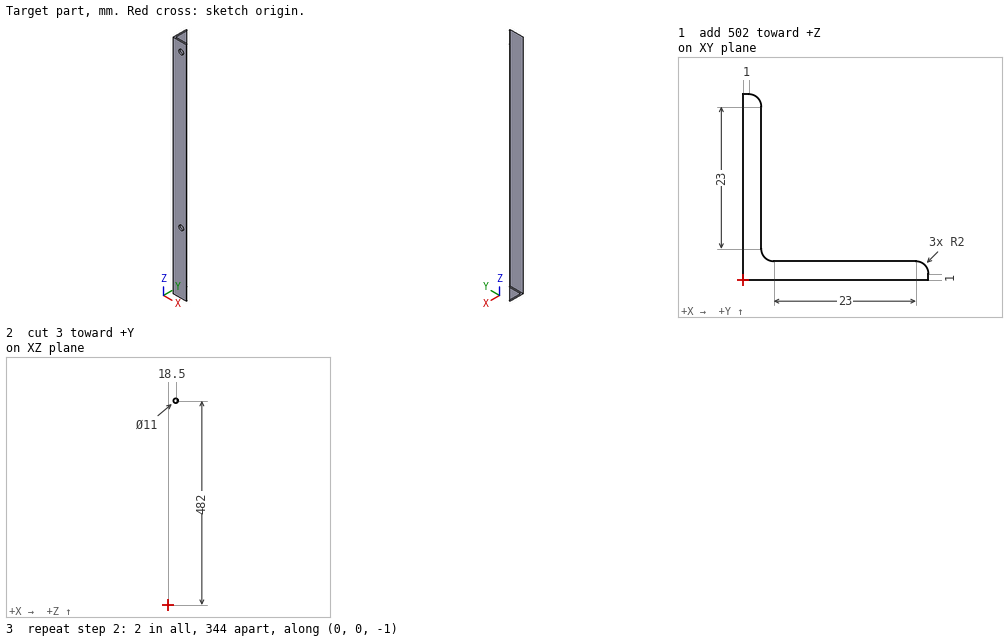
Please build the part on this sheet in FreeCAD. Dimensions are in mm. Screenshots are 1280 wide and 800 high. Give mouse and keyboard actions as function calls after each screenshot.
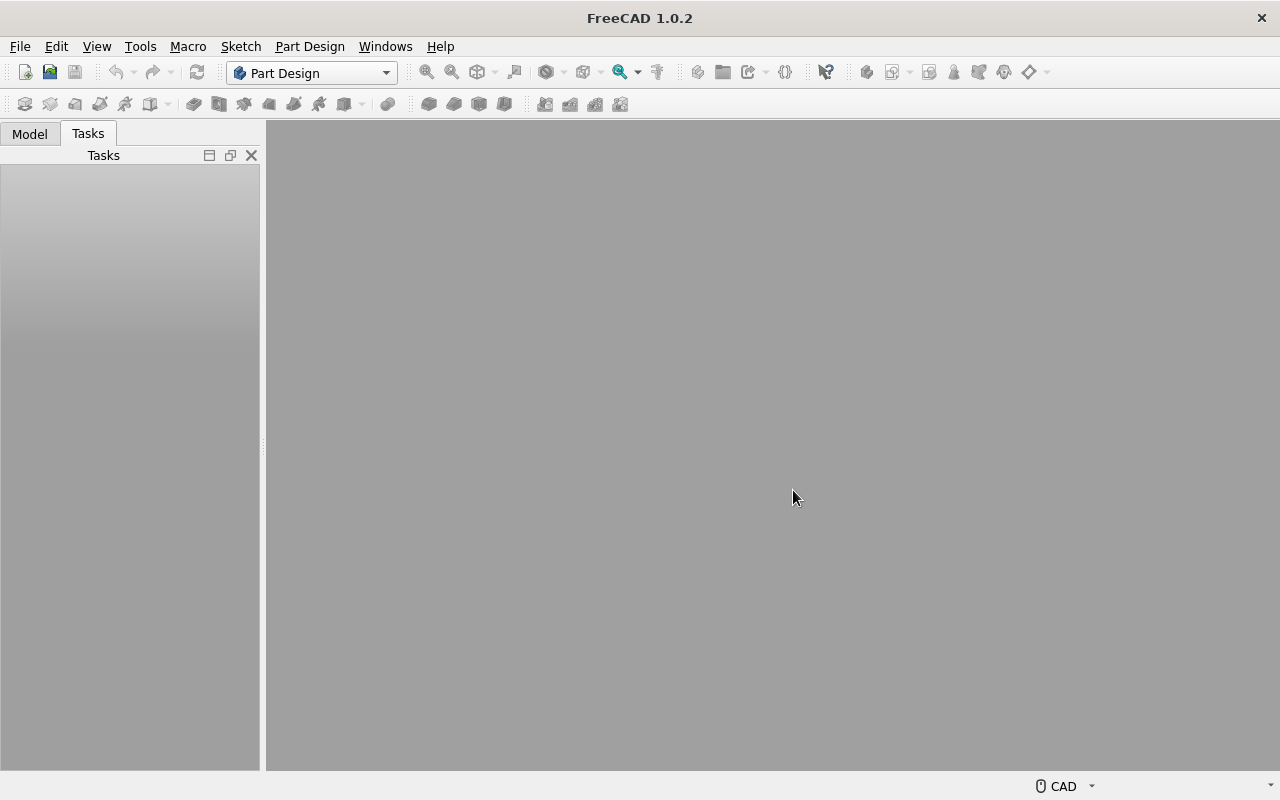
click(25, 72)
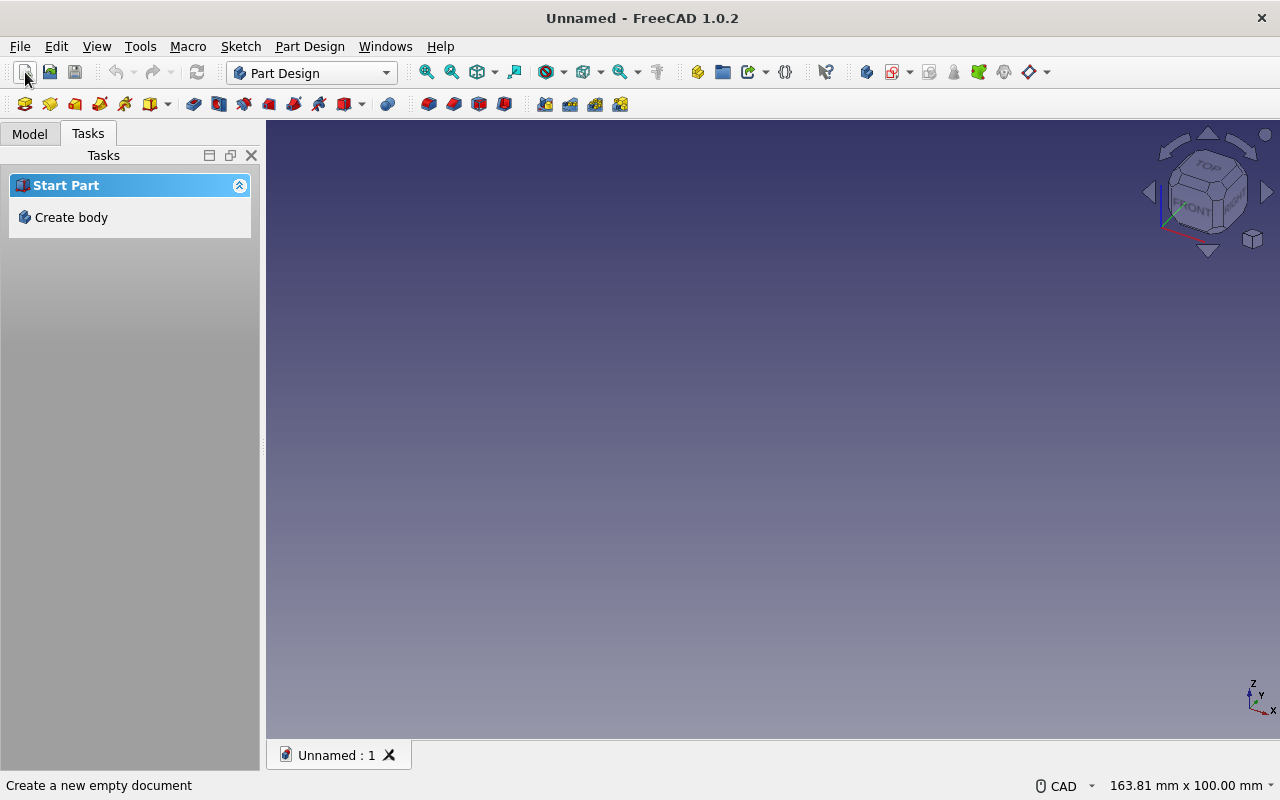
click(892, 72)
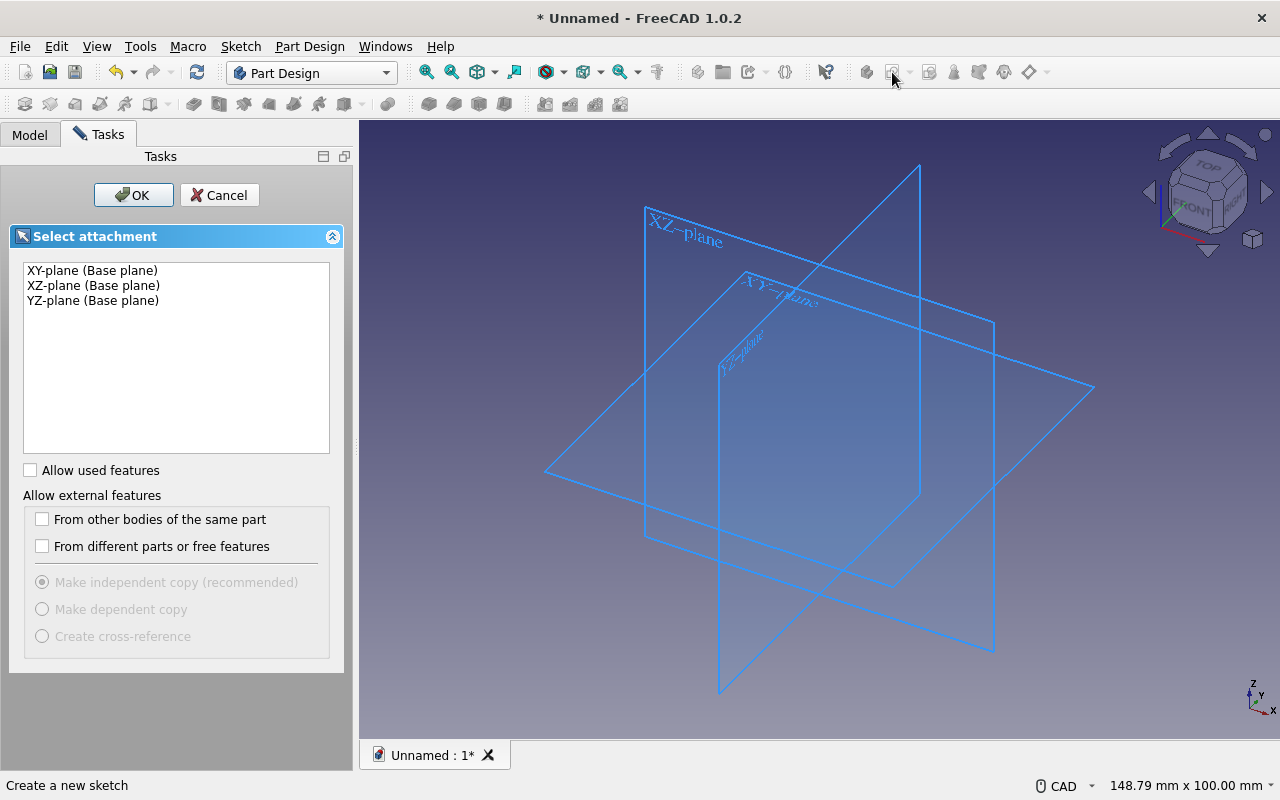
click(84, 270)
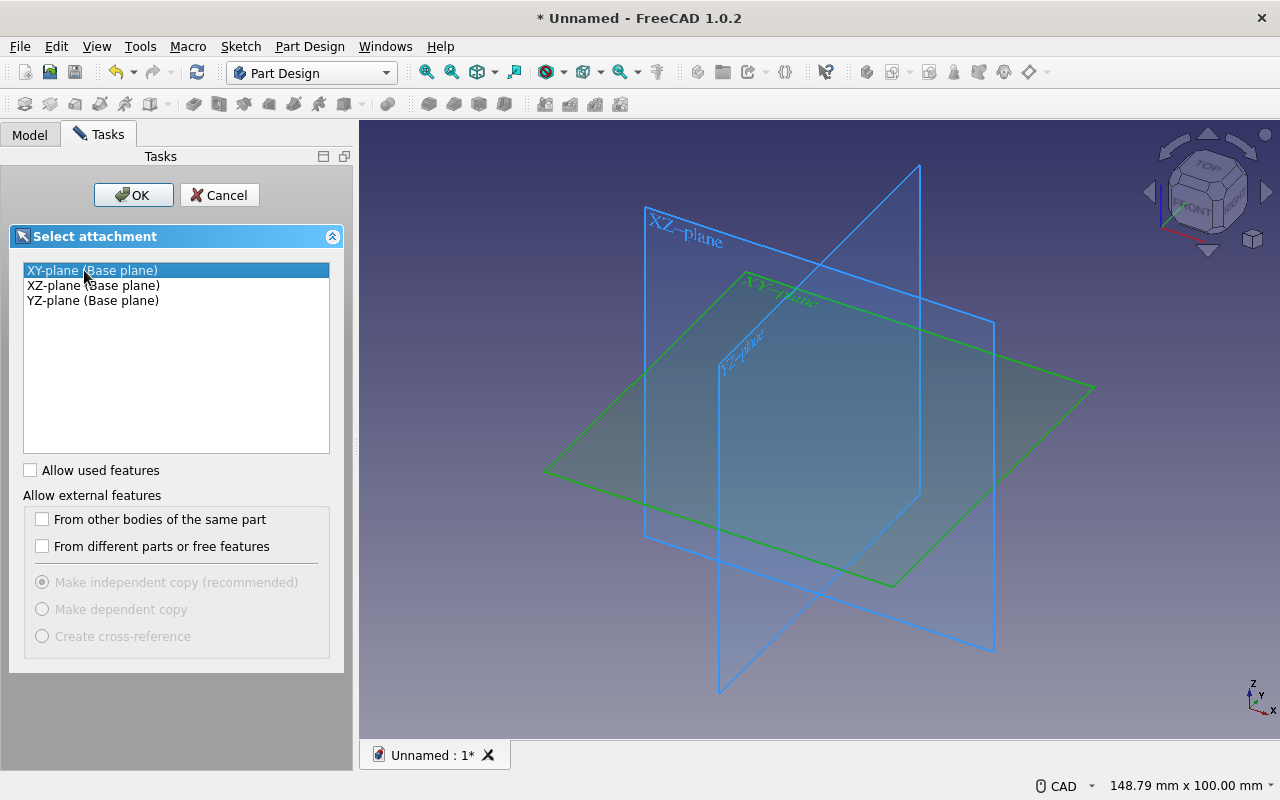
click(134, 195)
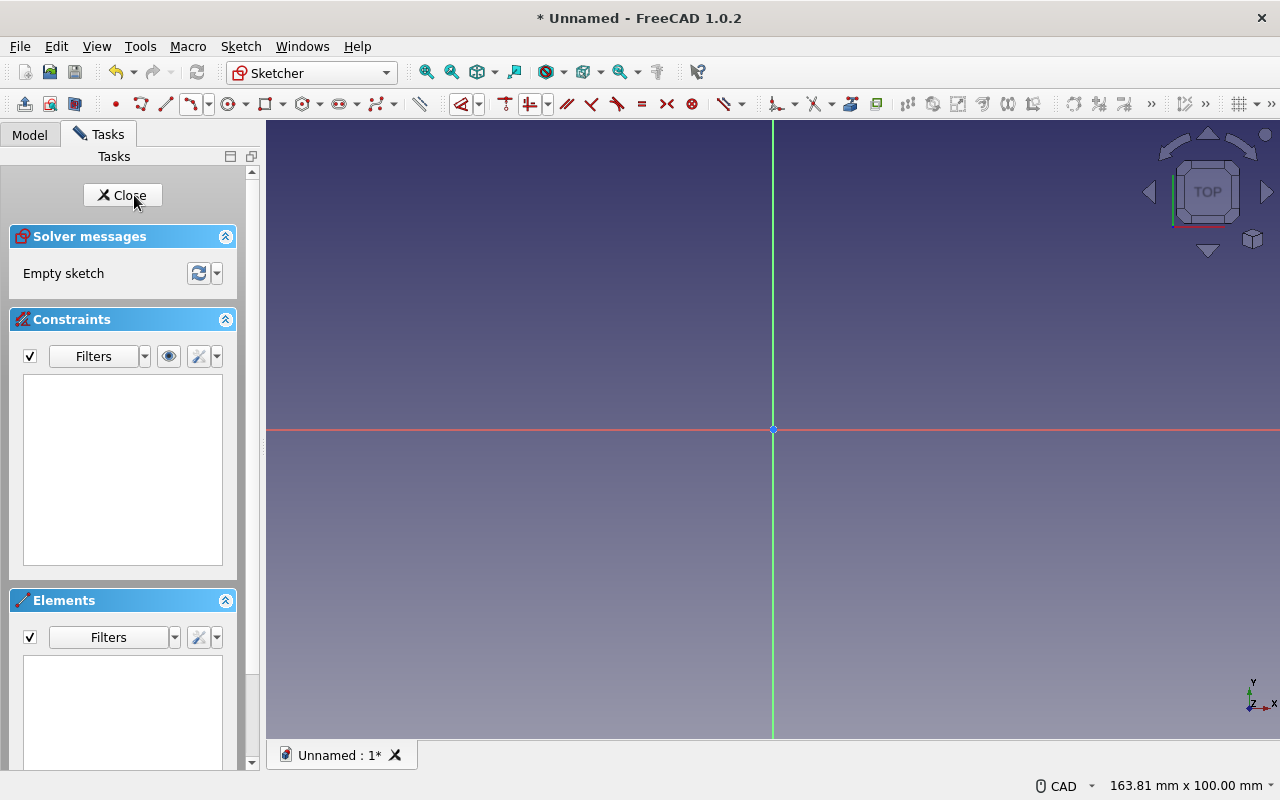
scroll(998, 261, up, 4)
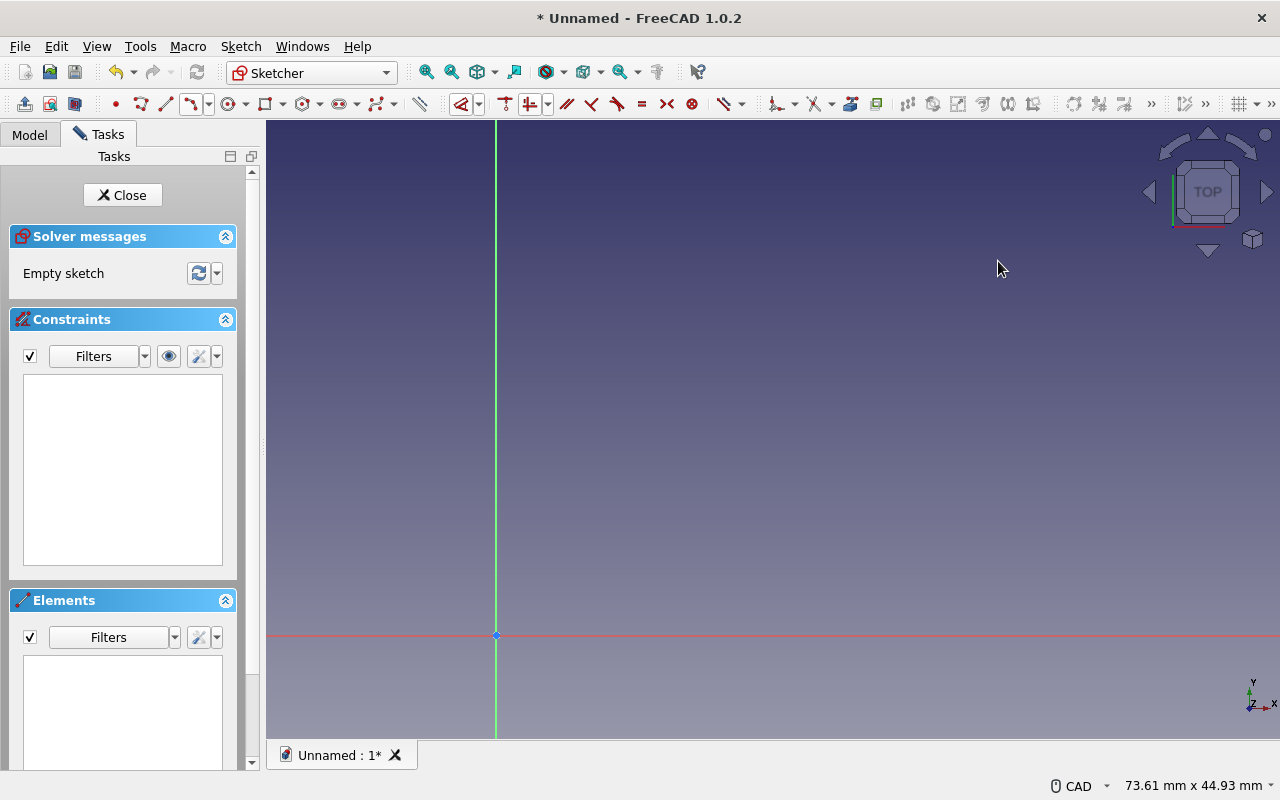
click(166, 104)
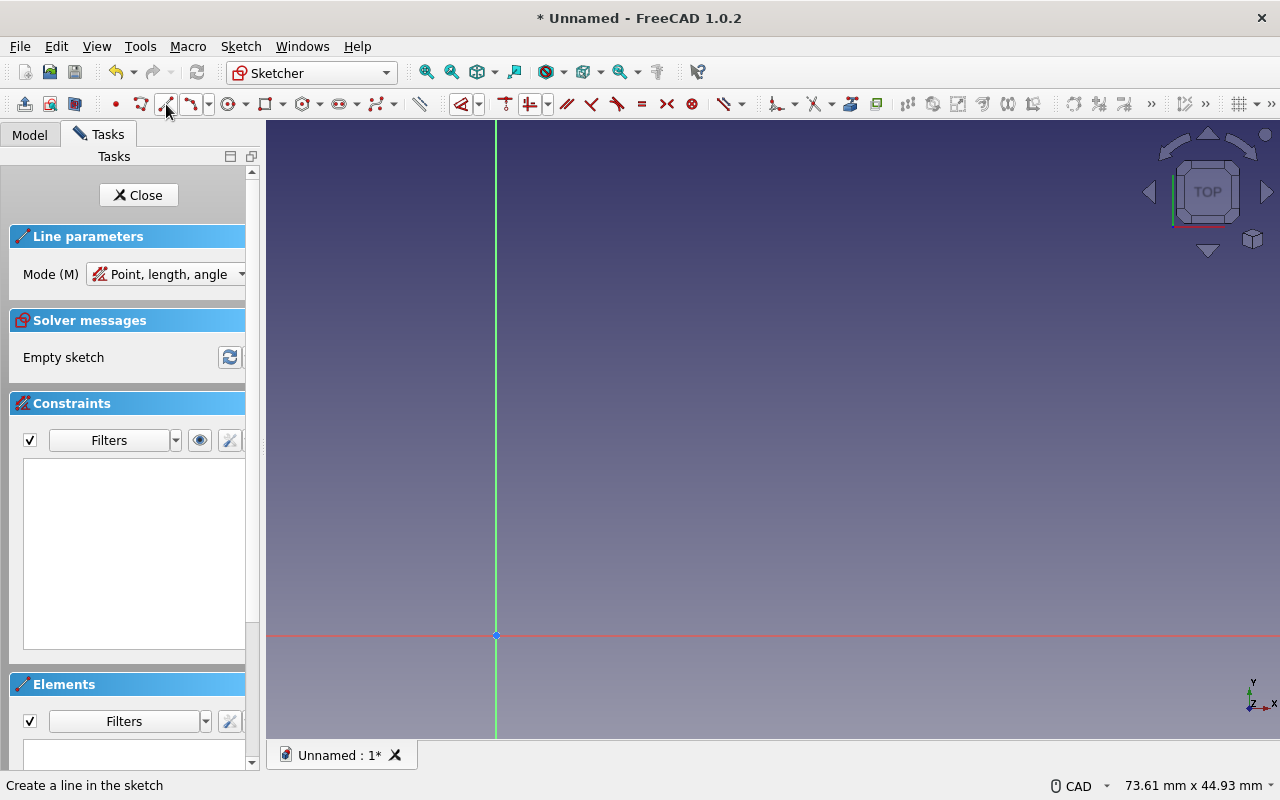
click(882, 594)
click(565, 594)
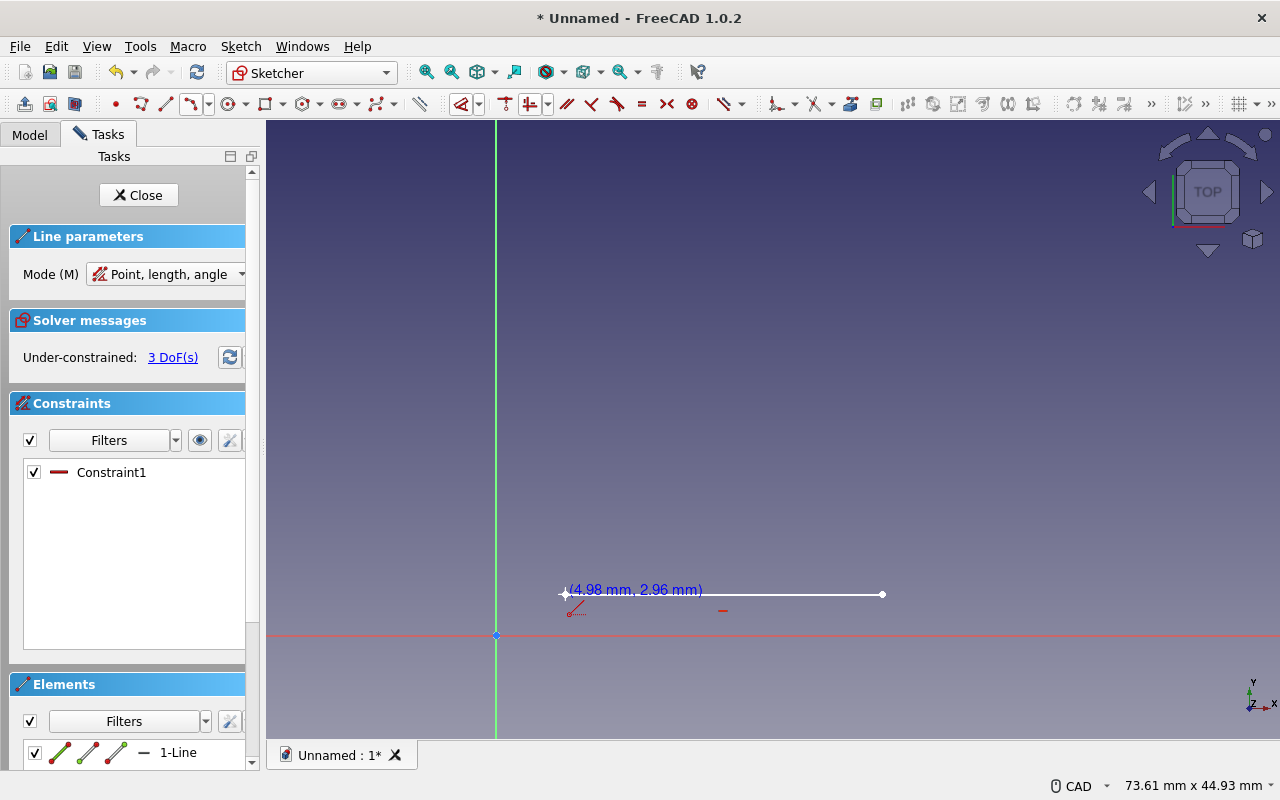
click(538, 567)
click(538, 250)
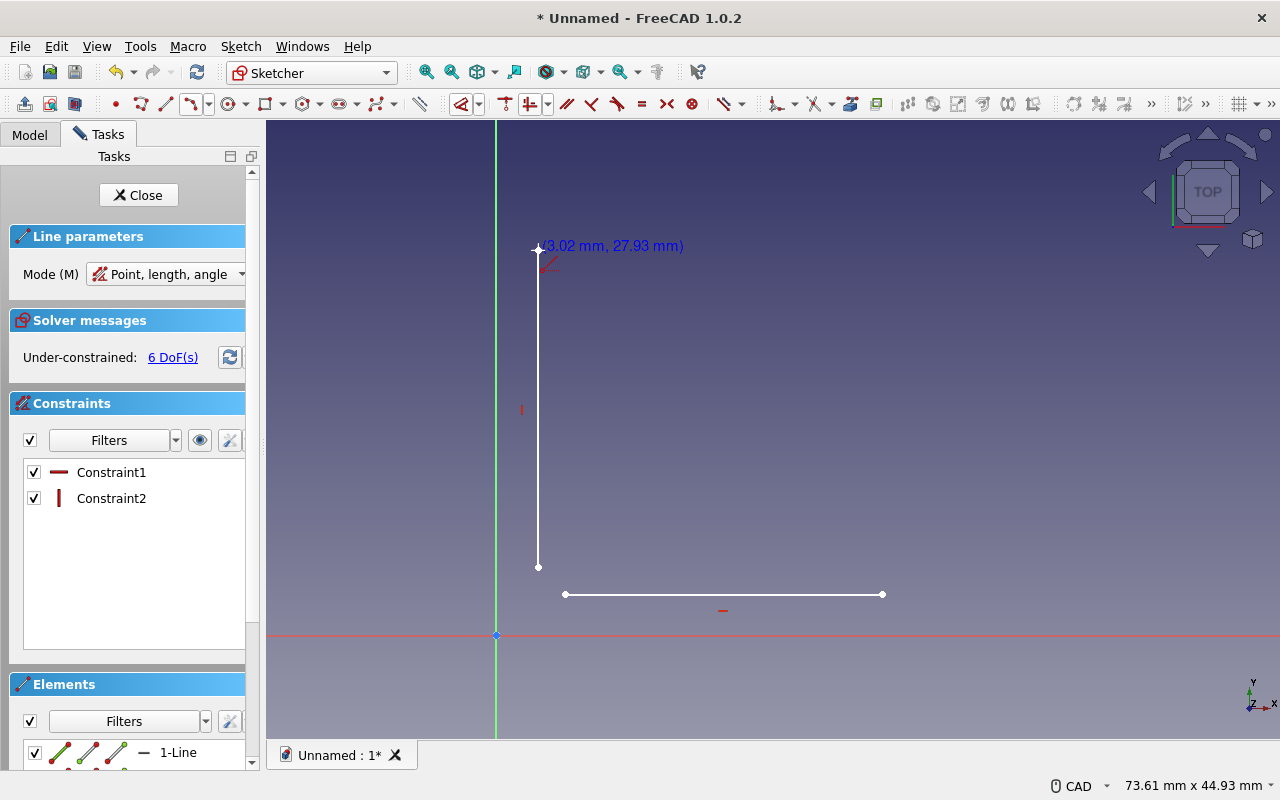
click(141, 104)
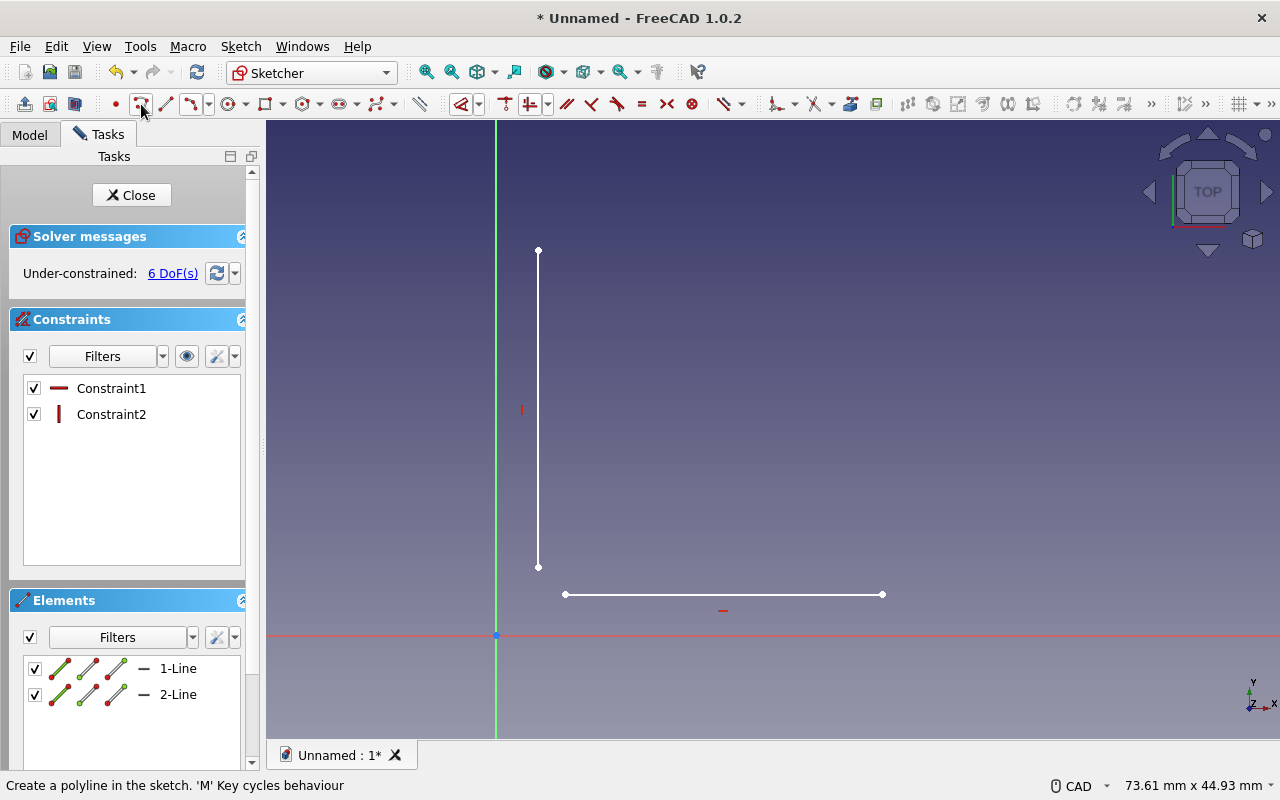
click(510, 222)
click(496, 222)
click(496, 636)
click(910, 627)
click(910, 622)
right_click(910, 622)